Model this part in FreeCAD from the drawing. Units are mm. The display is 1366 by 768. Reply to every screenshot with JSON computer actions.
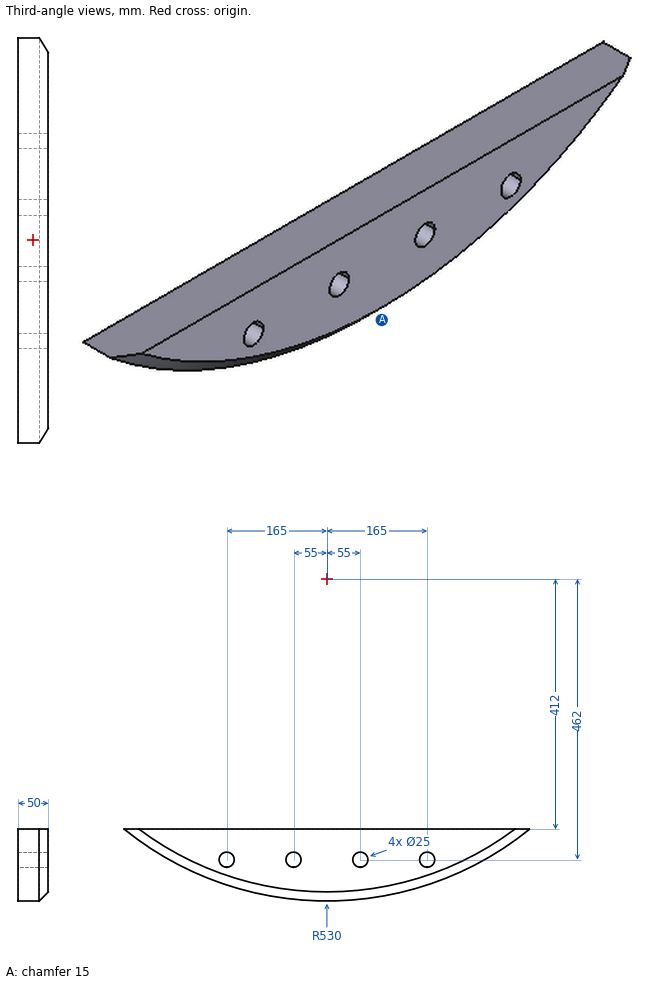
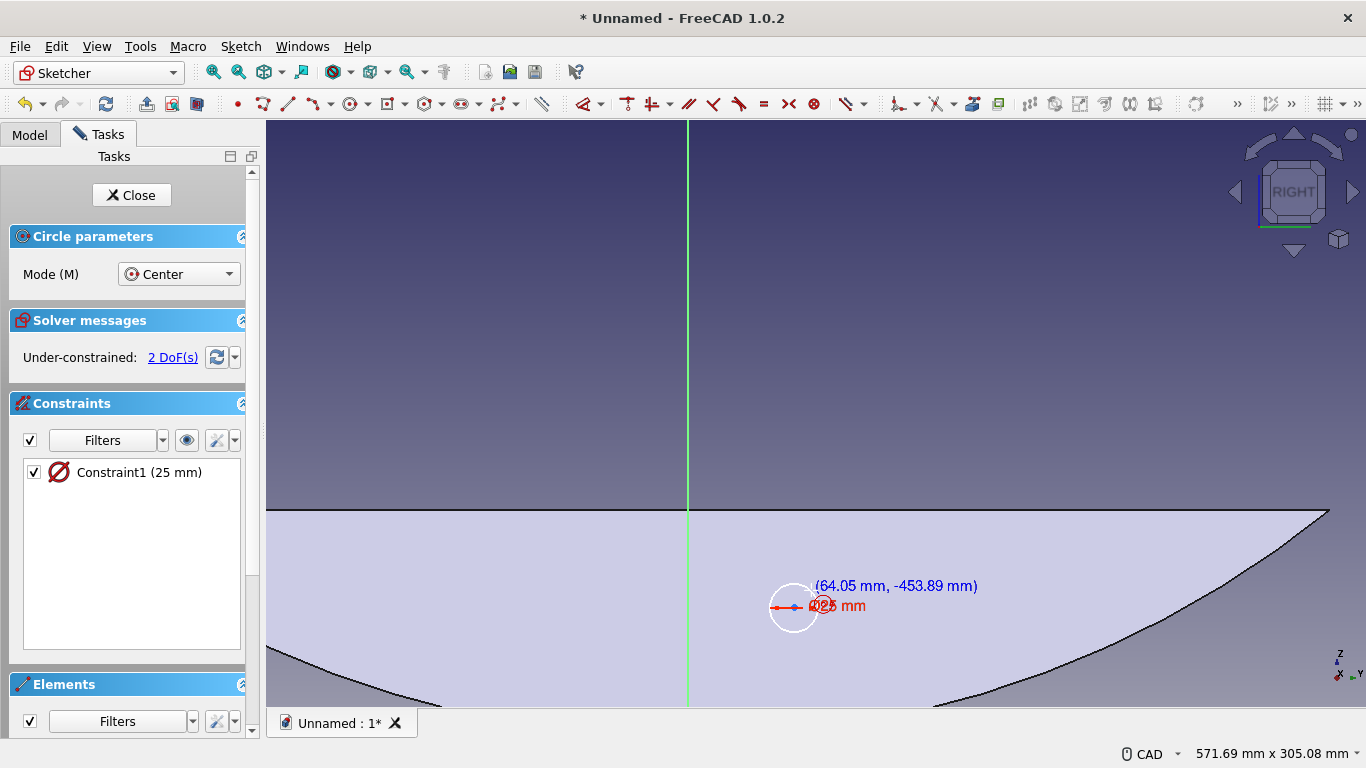
{"action": "left_click", "coordinate": [582, 607]}
{"action": "mouse_move", "coordinate": [599, 590]}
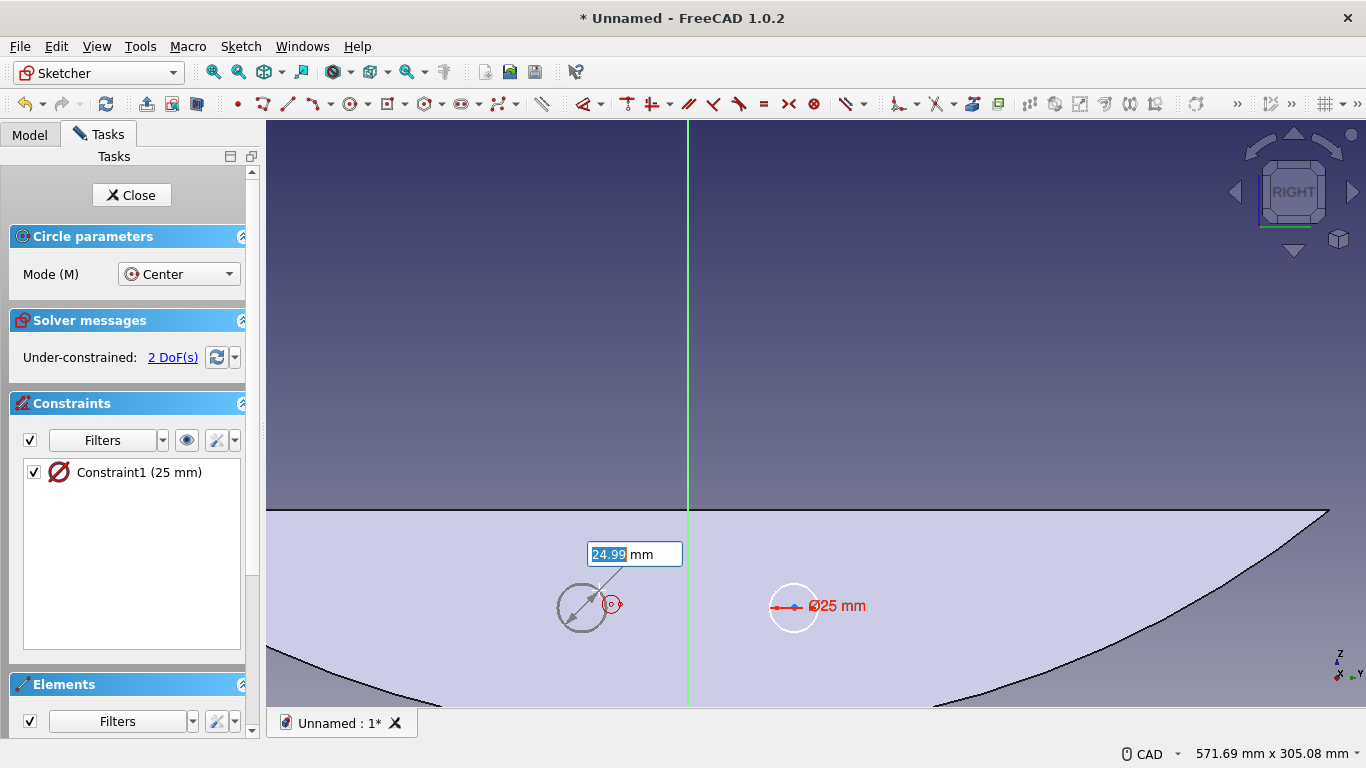
{"action": "type", "text": "25"}
{"action": "key", "text": "Return"}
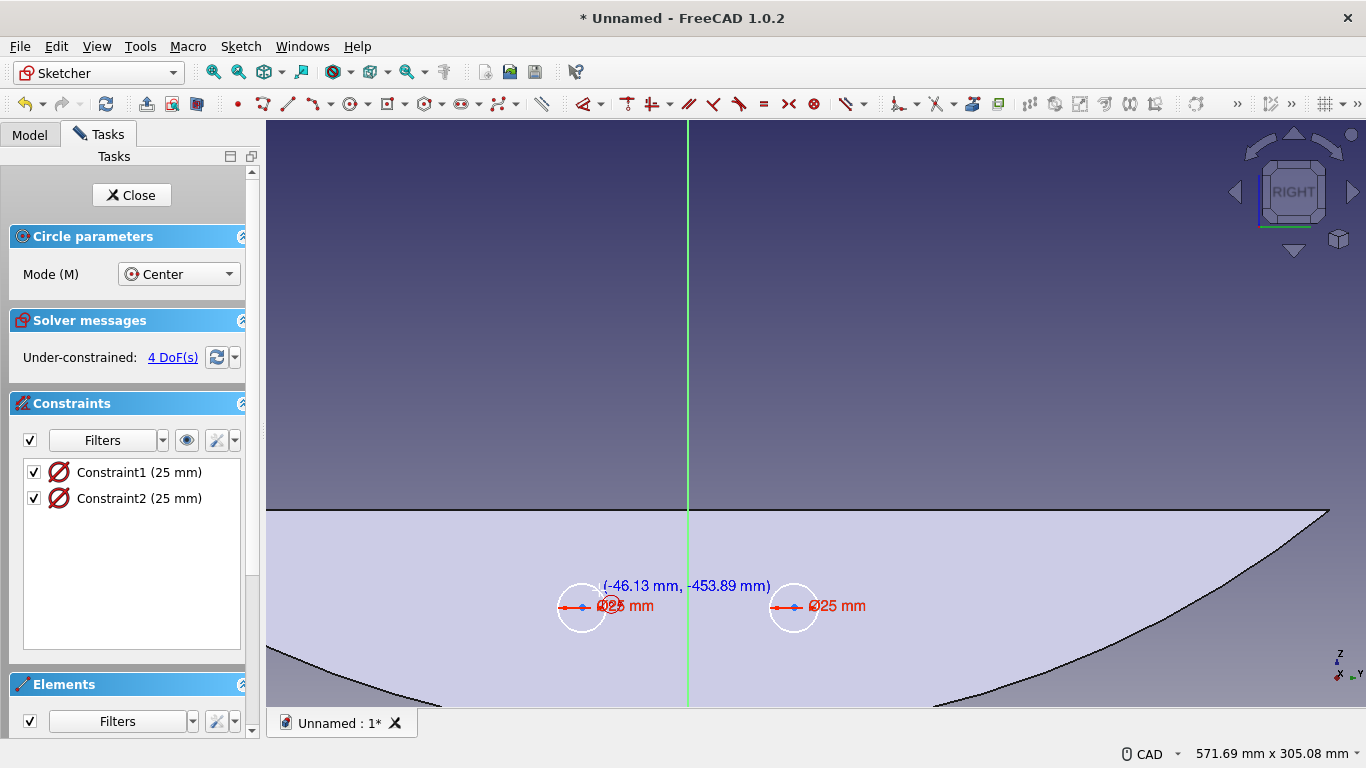
{"action": "left_click", "coordinate": [1005, 607]}
{"action": "mouse_move", "coordinate": [1022, 590]}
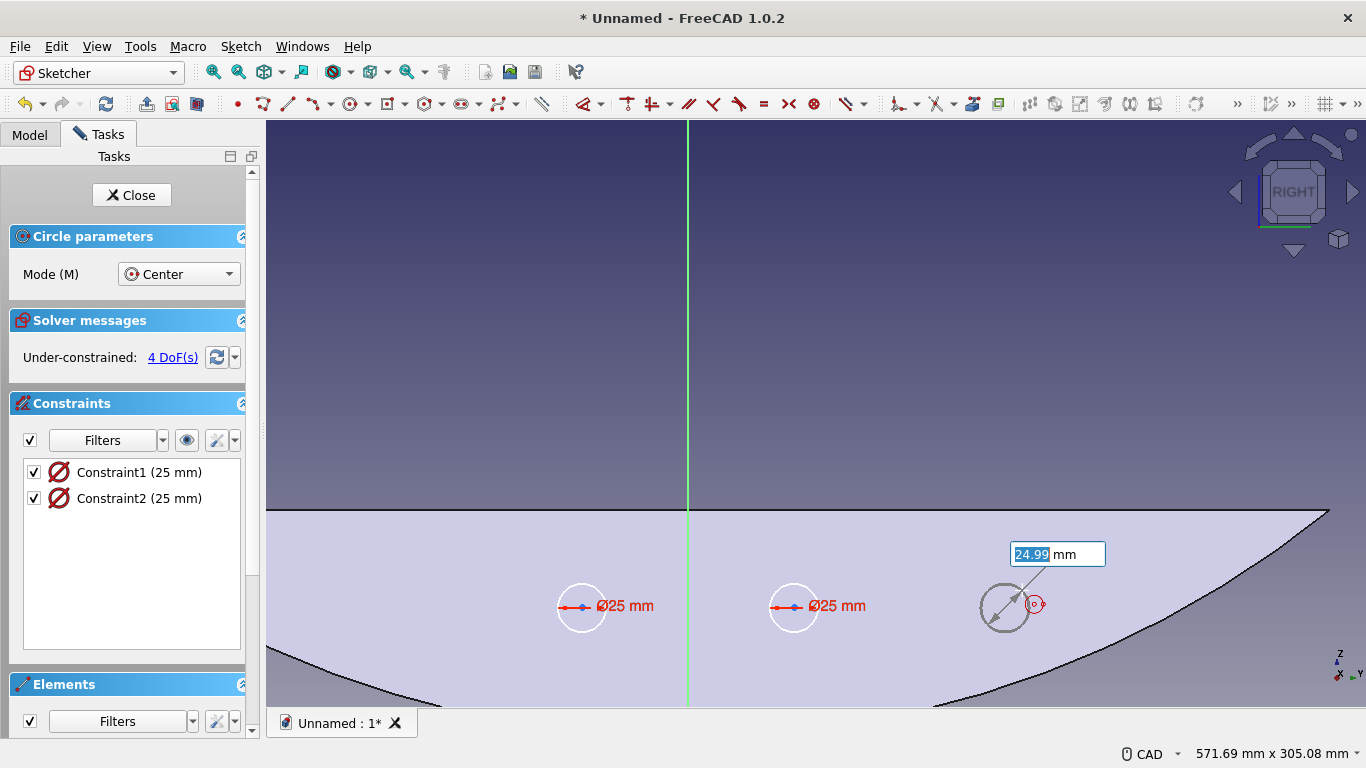
{"action": "type", "text": "25"}
{"action": "key", "text": "Return"}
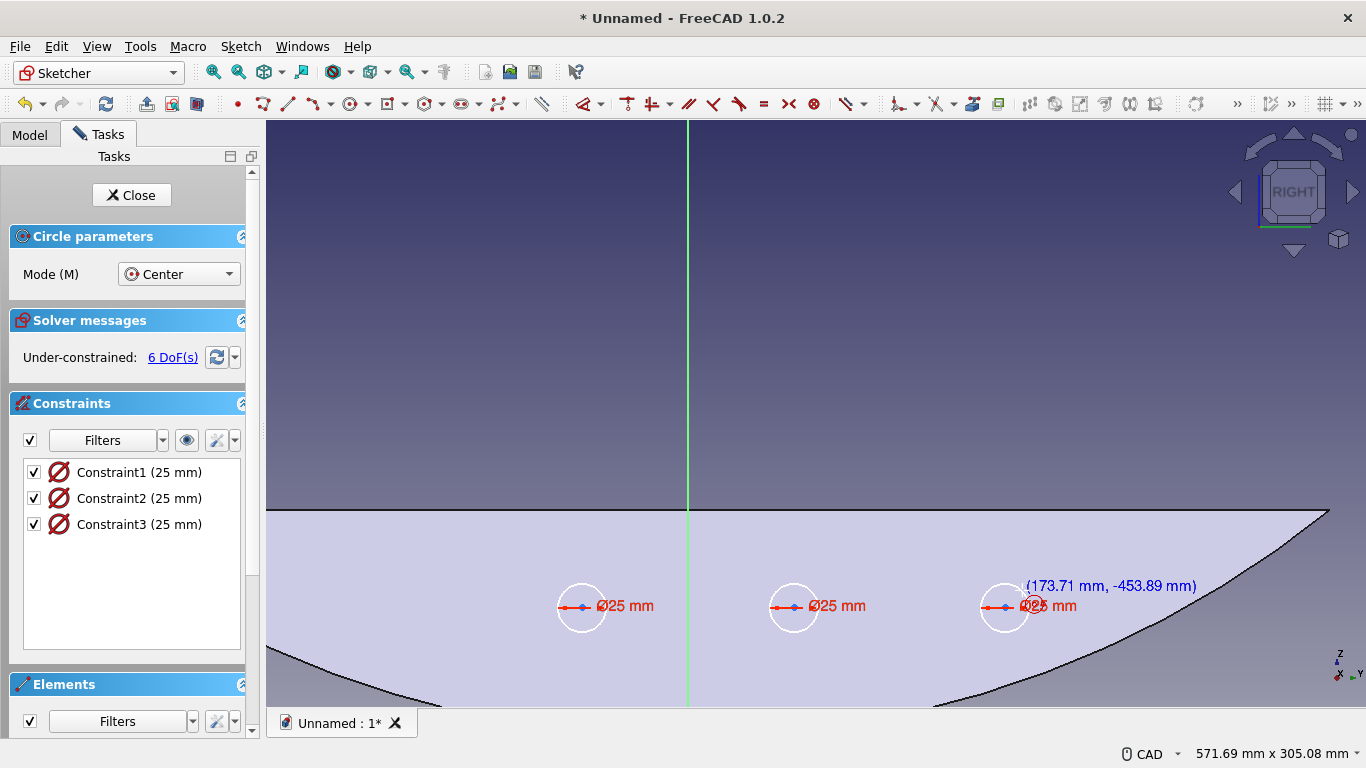
{"action": "left_click", "coordinate": [370, 607]}
{"action": "mouse_move", "coordinate": [387, 590]}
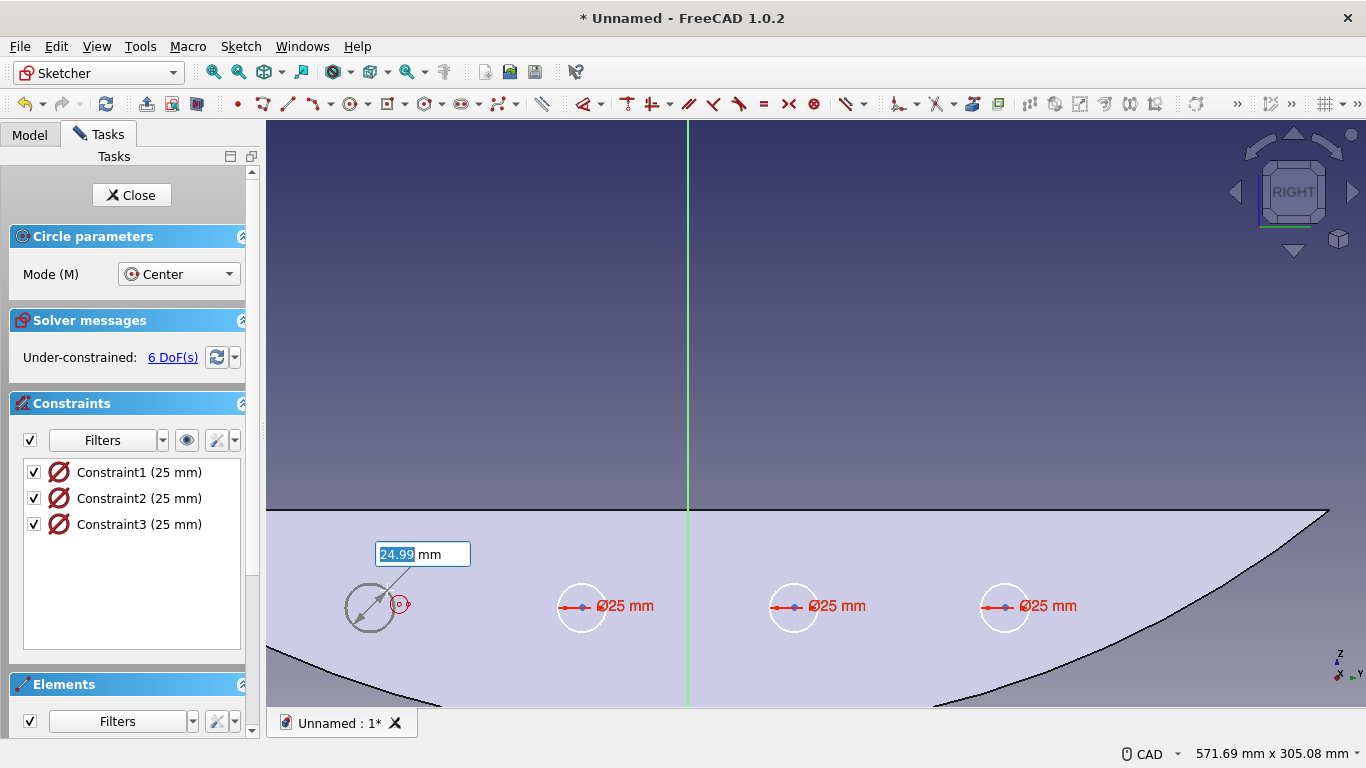
{"action": "type", "text": "25"}
{"action": "key", "text": "Return"}
{"action": "key", "text": "Escape"}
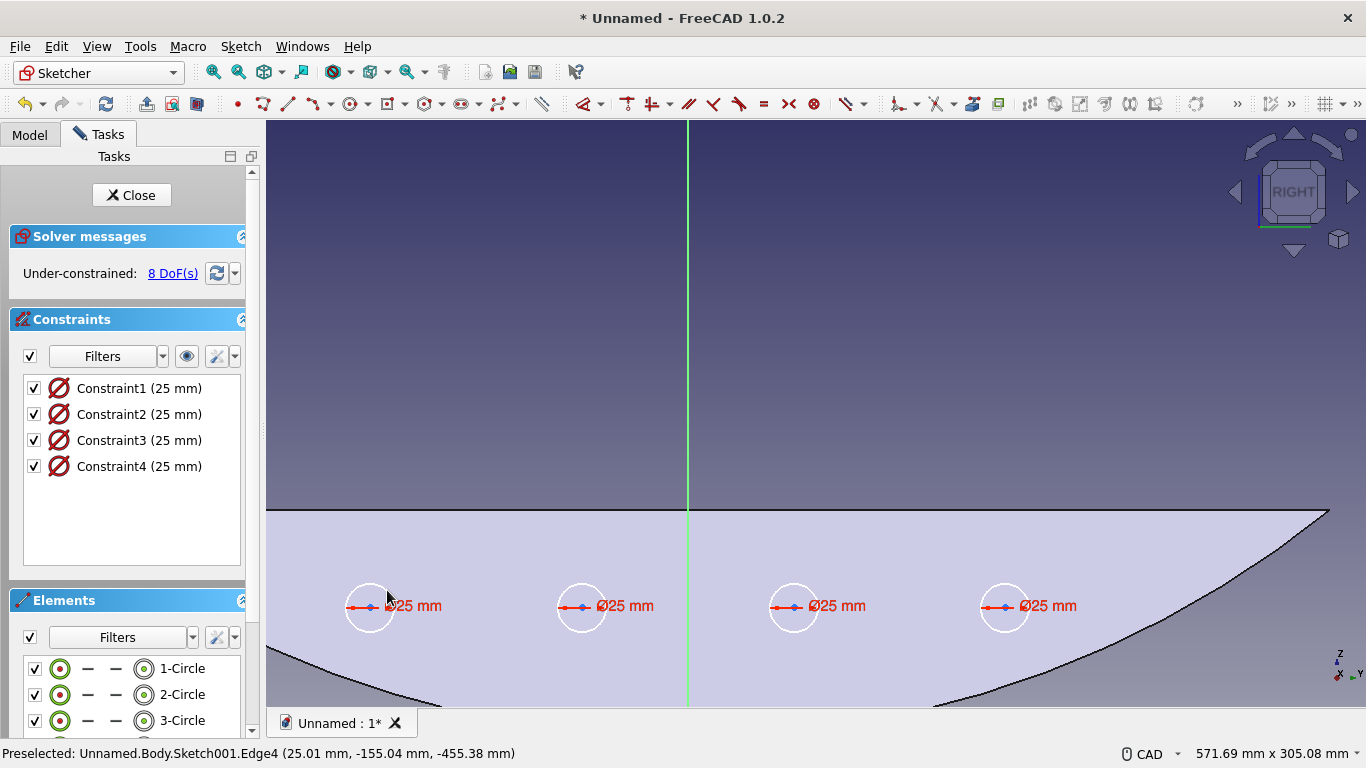
{"action": "left_click", "coordinate": [794, 608]}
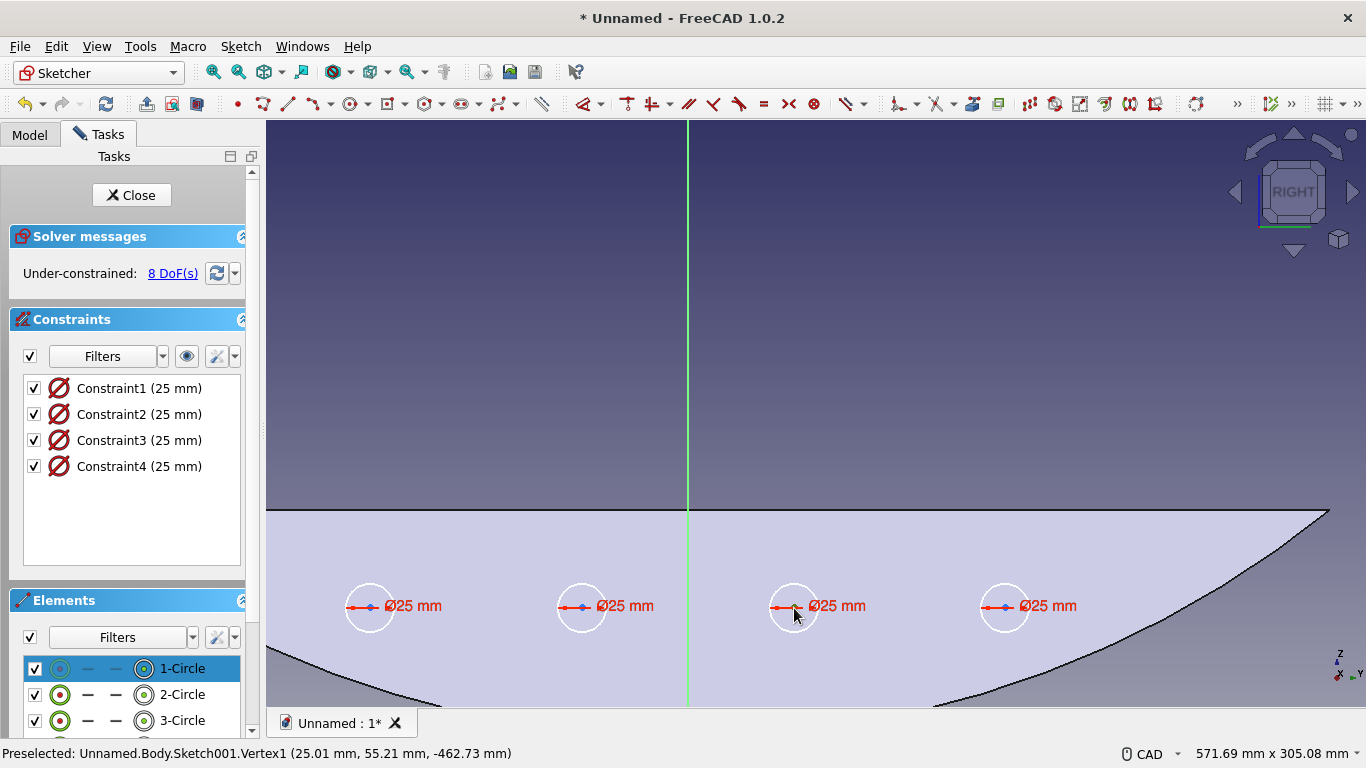
{"action": "left_click", "coordinate": [582, 608]}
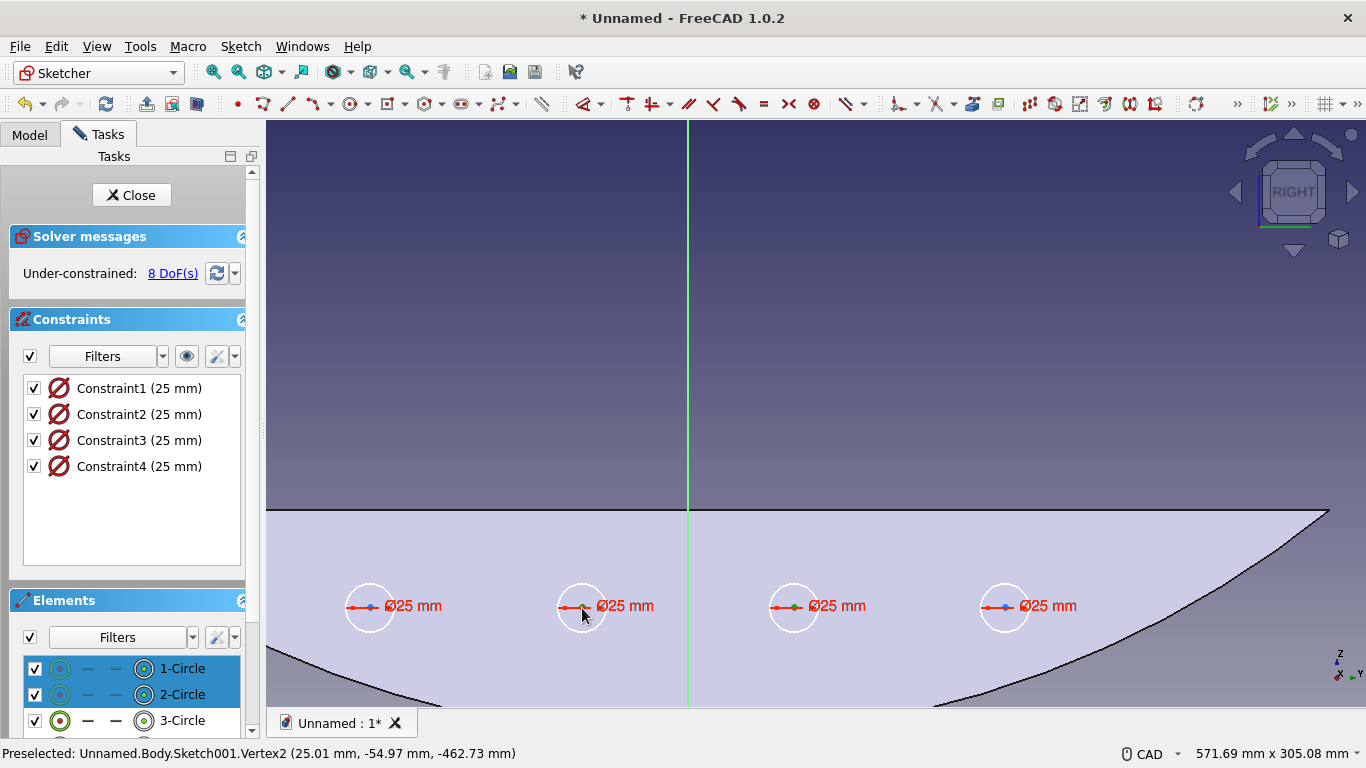
{"action": "key", "text": "h"}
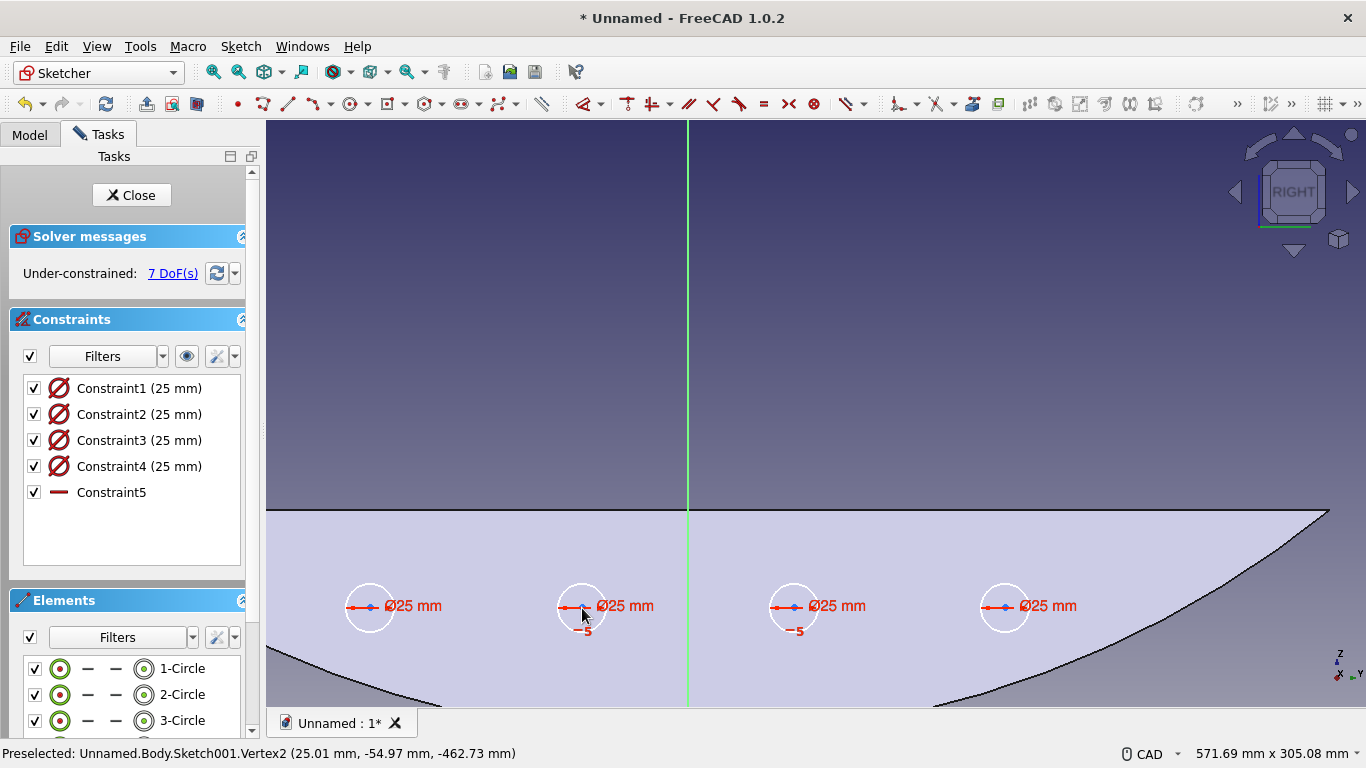
{"action": "left_click", "coordinate": [794, 608]}